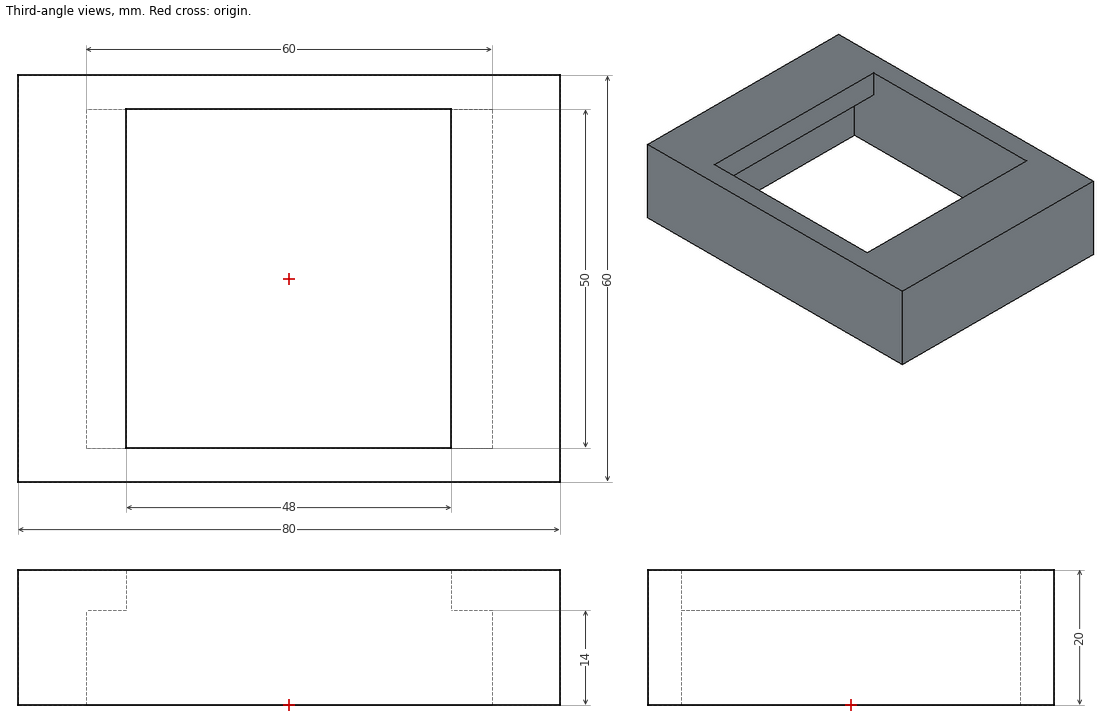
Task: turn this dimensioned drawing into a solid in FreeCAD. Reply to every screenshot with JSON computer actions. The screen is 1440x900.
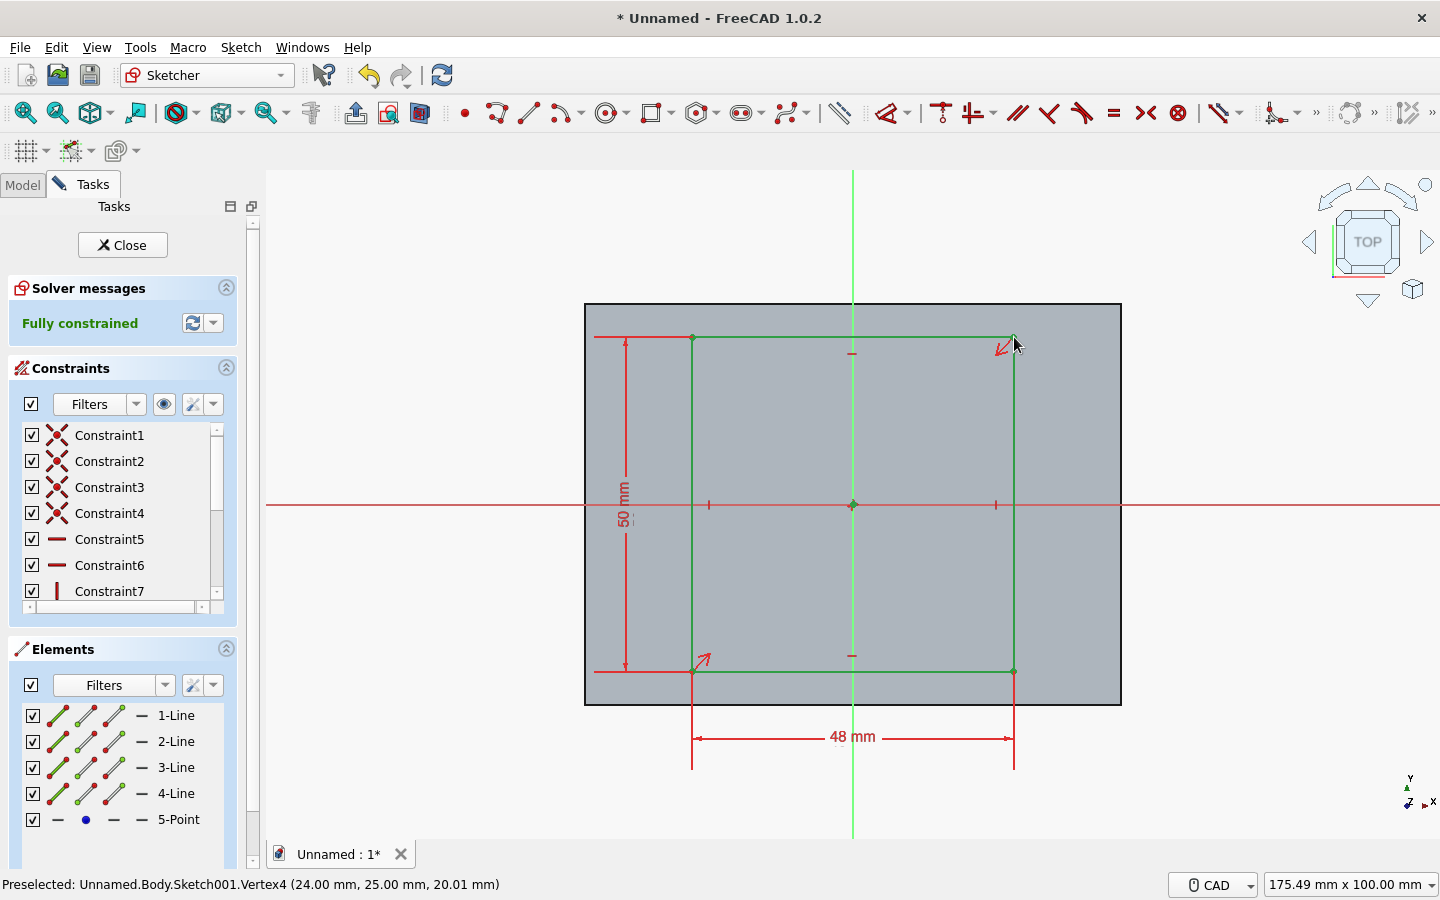
{"action": "left_click", "coordinate": [123, 245]}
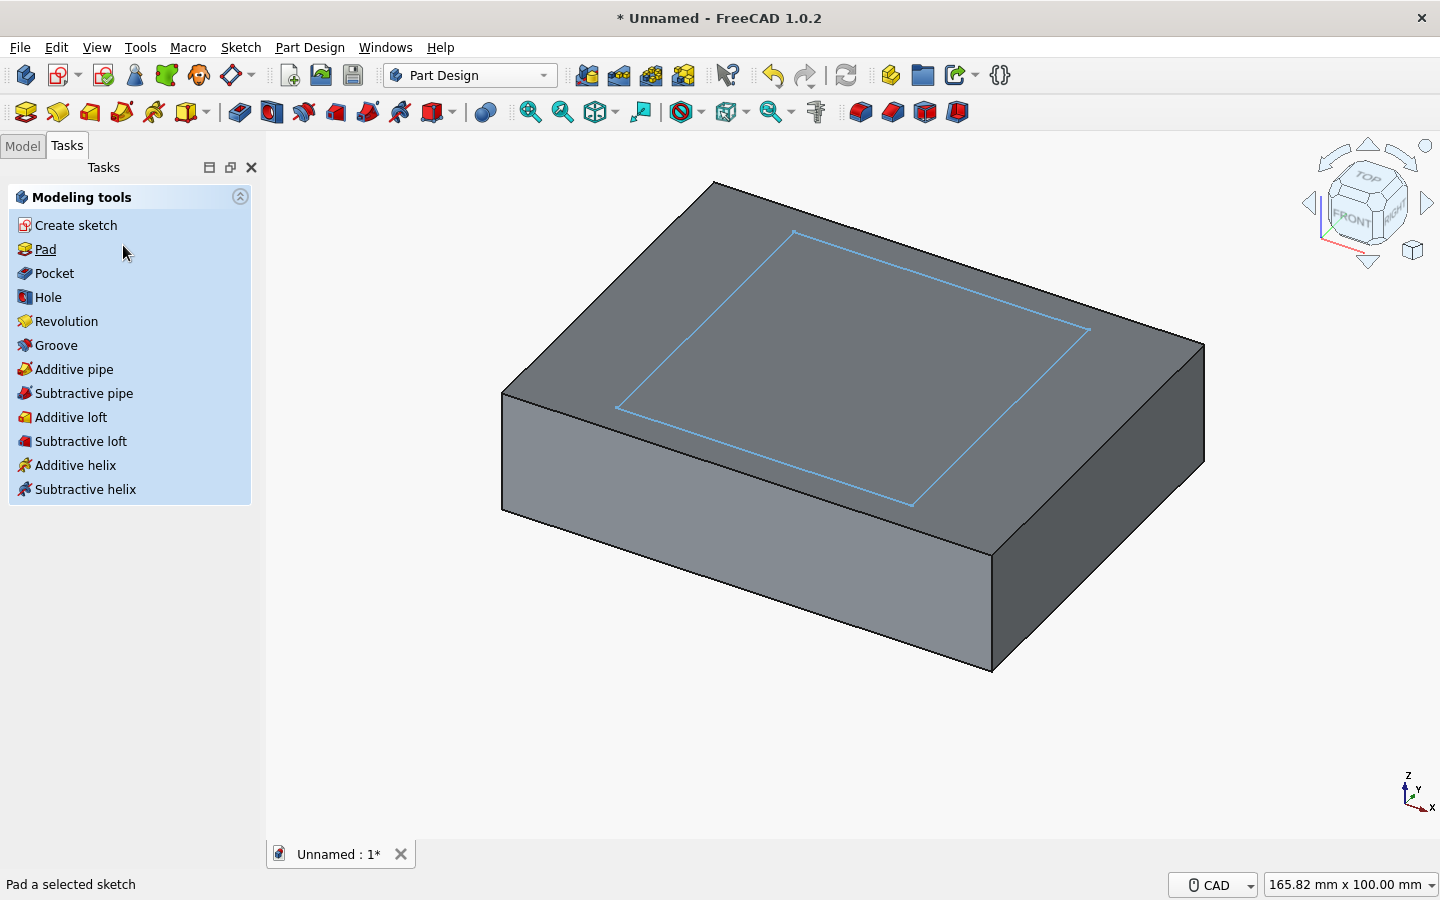
{"action": "left_click", "coordinate": [240, 112]}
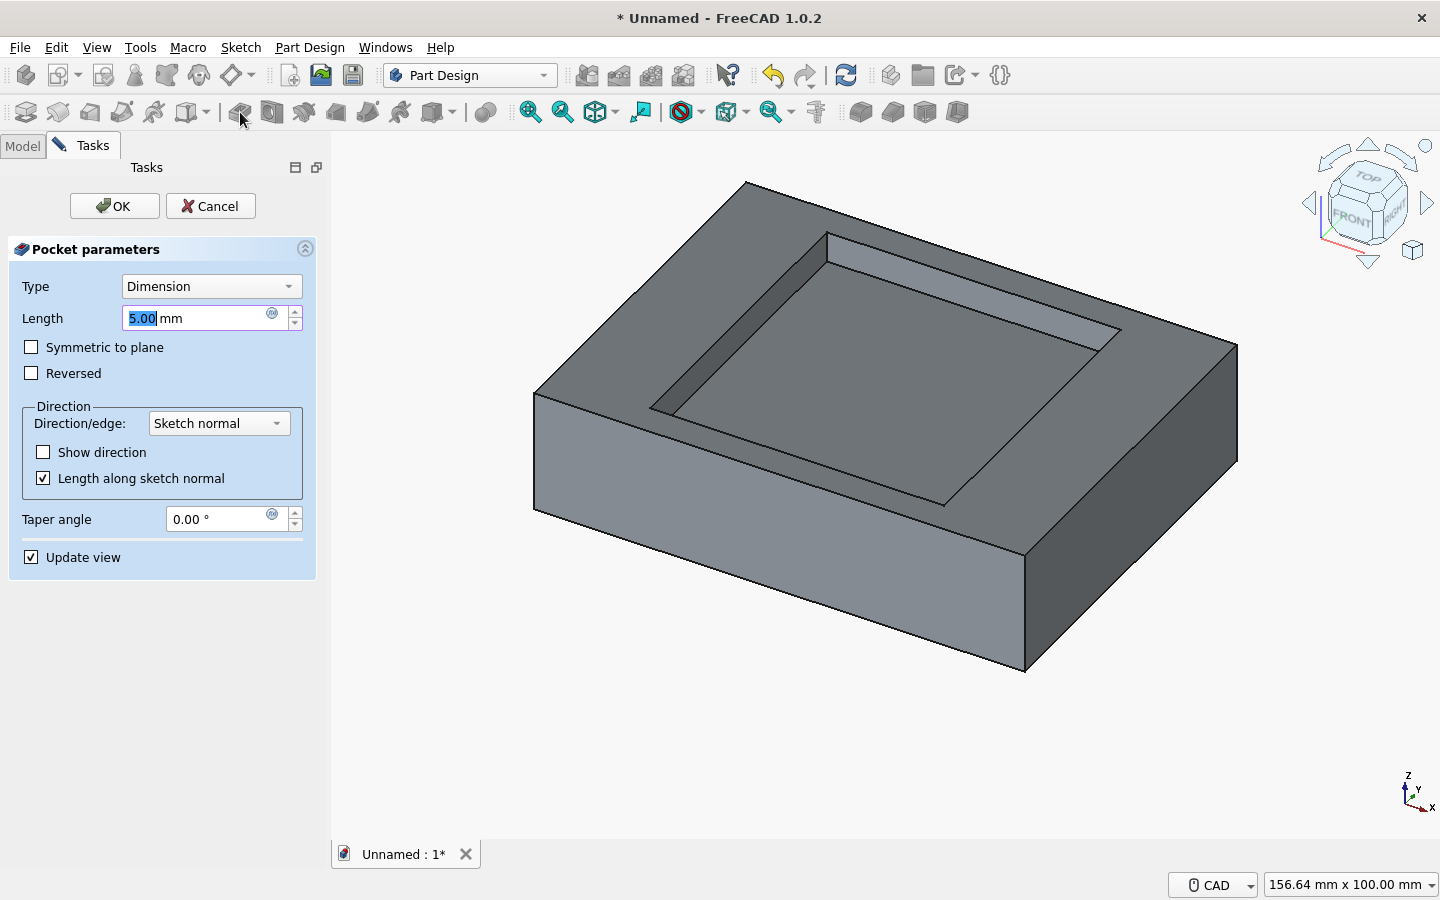
{"action": "left_click", "coordinate": [212, 286]}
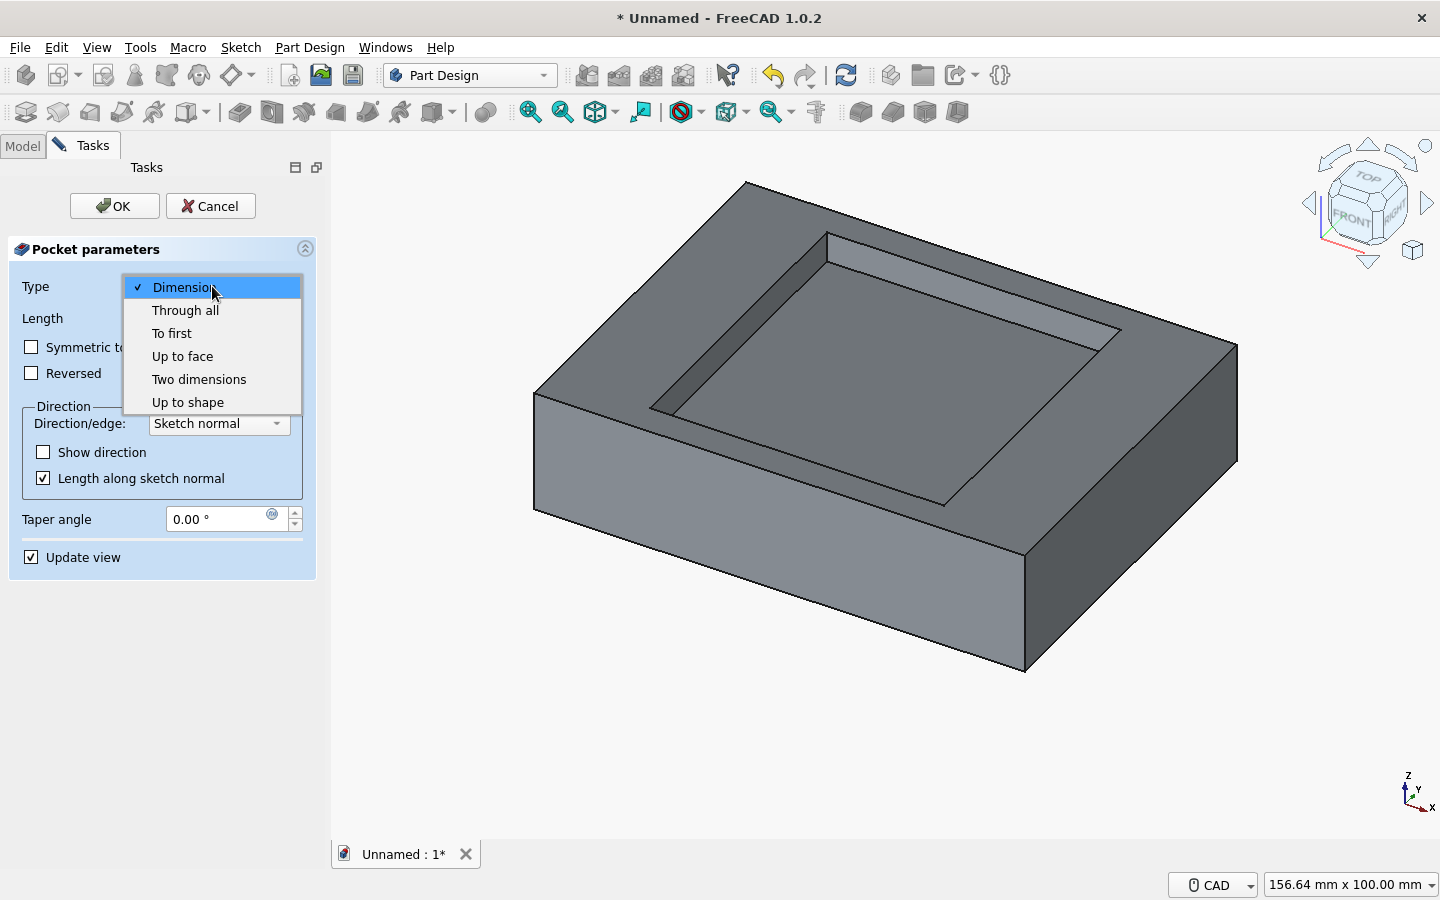
{"action": "left_click", "coordinate": [212, 334]}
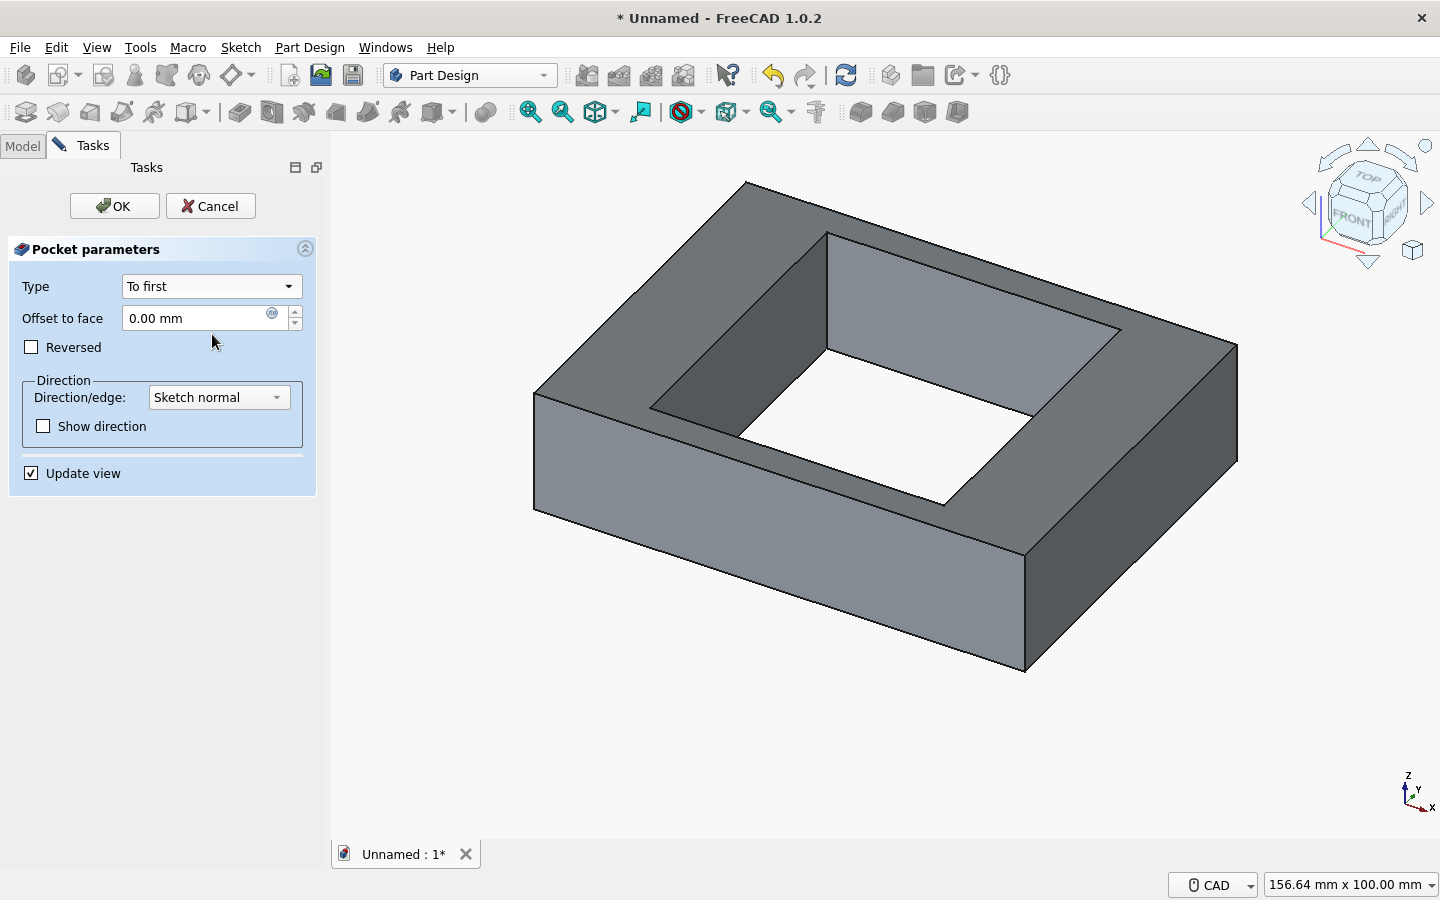
{"action": "left_click", "coordinate": [115, 206]}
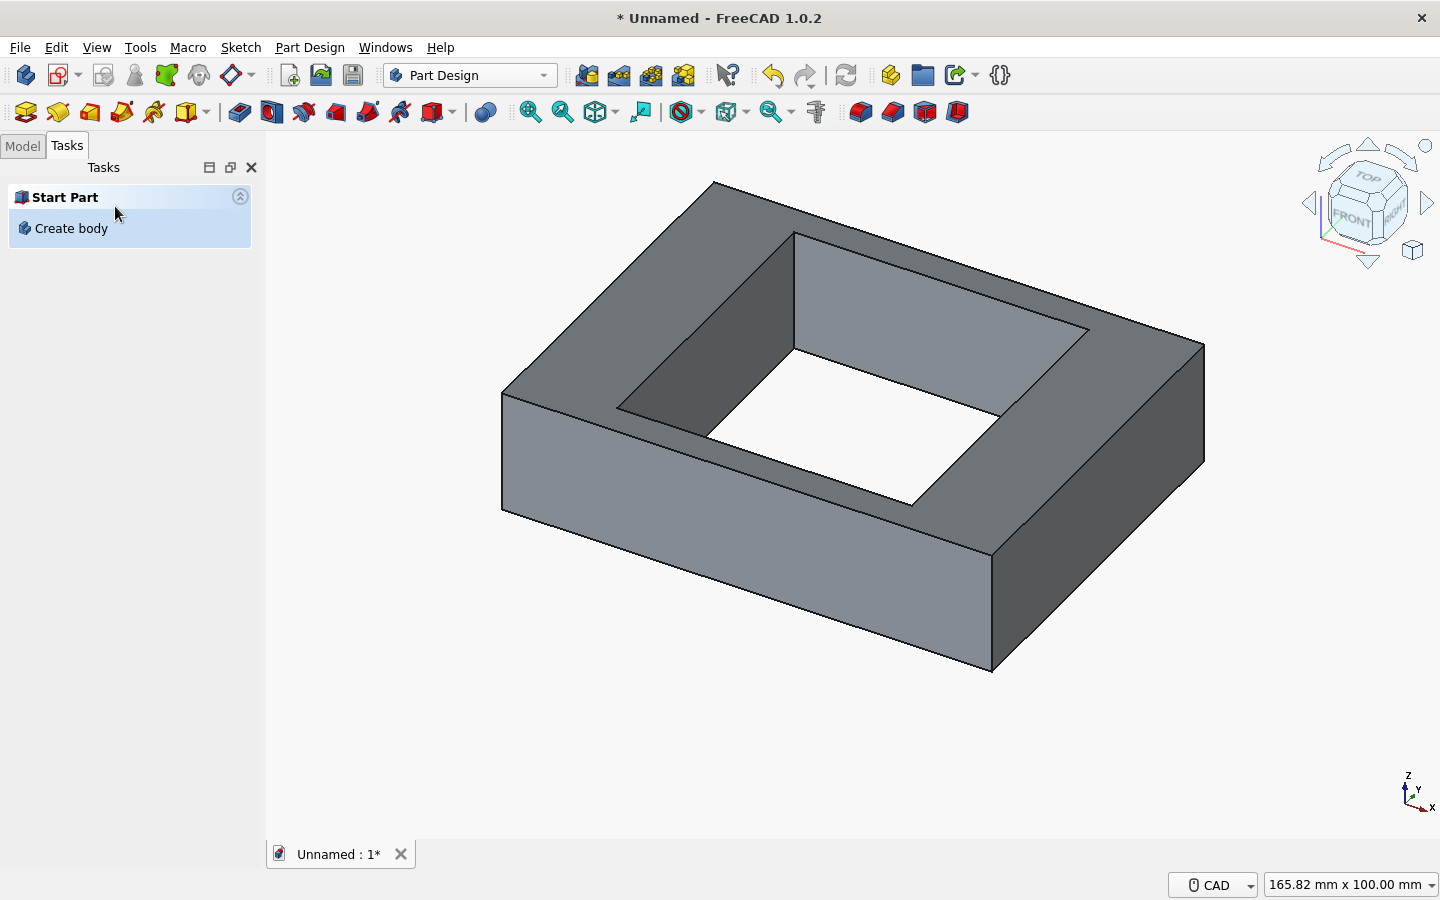
{"action": "key", "text": "5"}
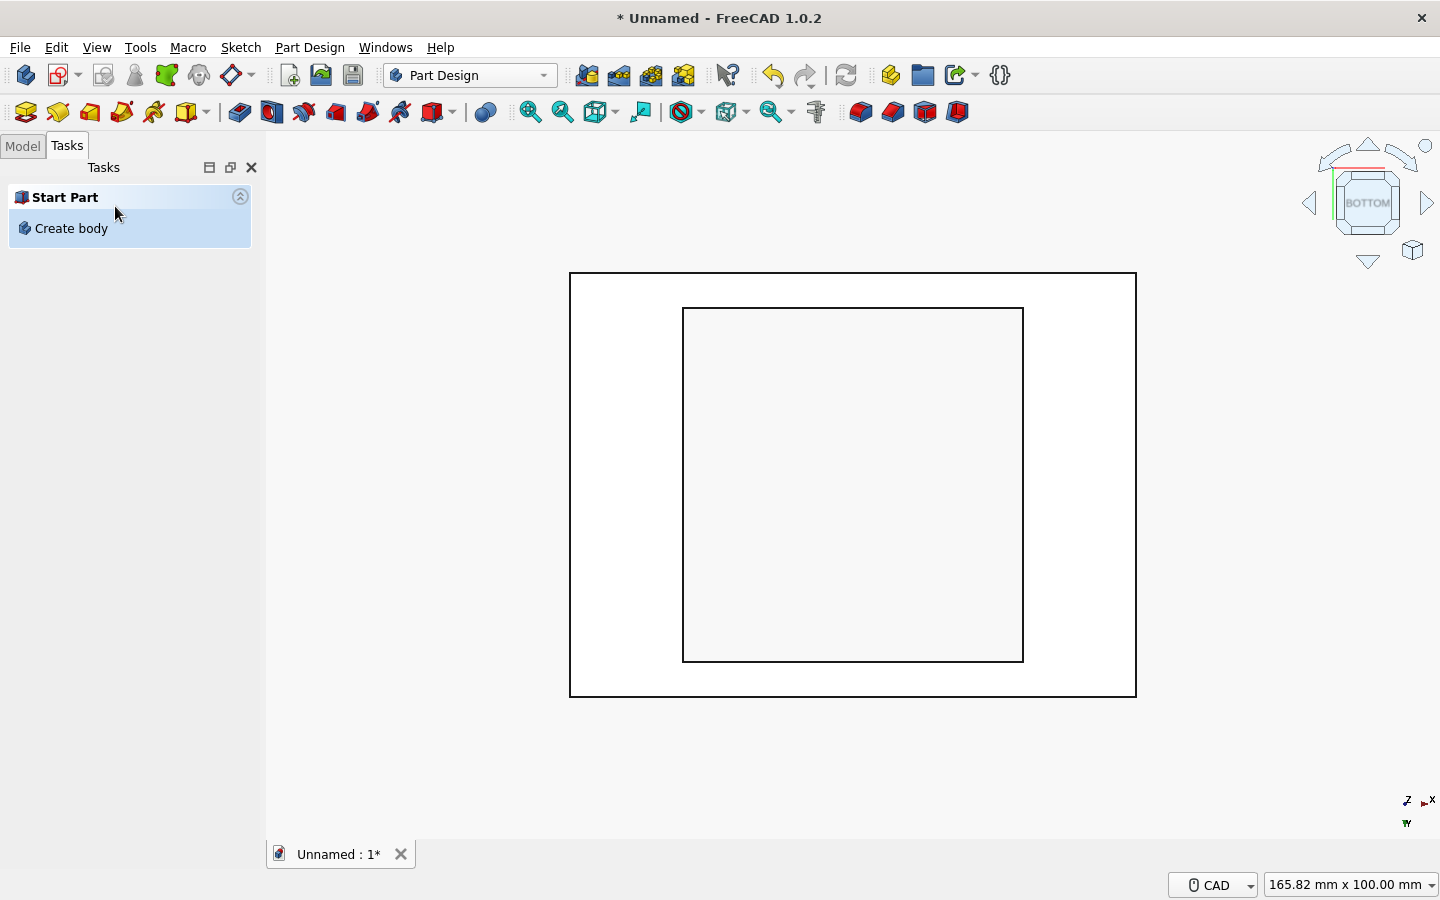
{"action": "left_click", "coordinate": [610, 605]}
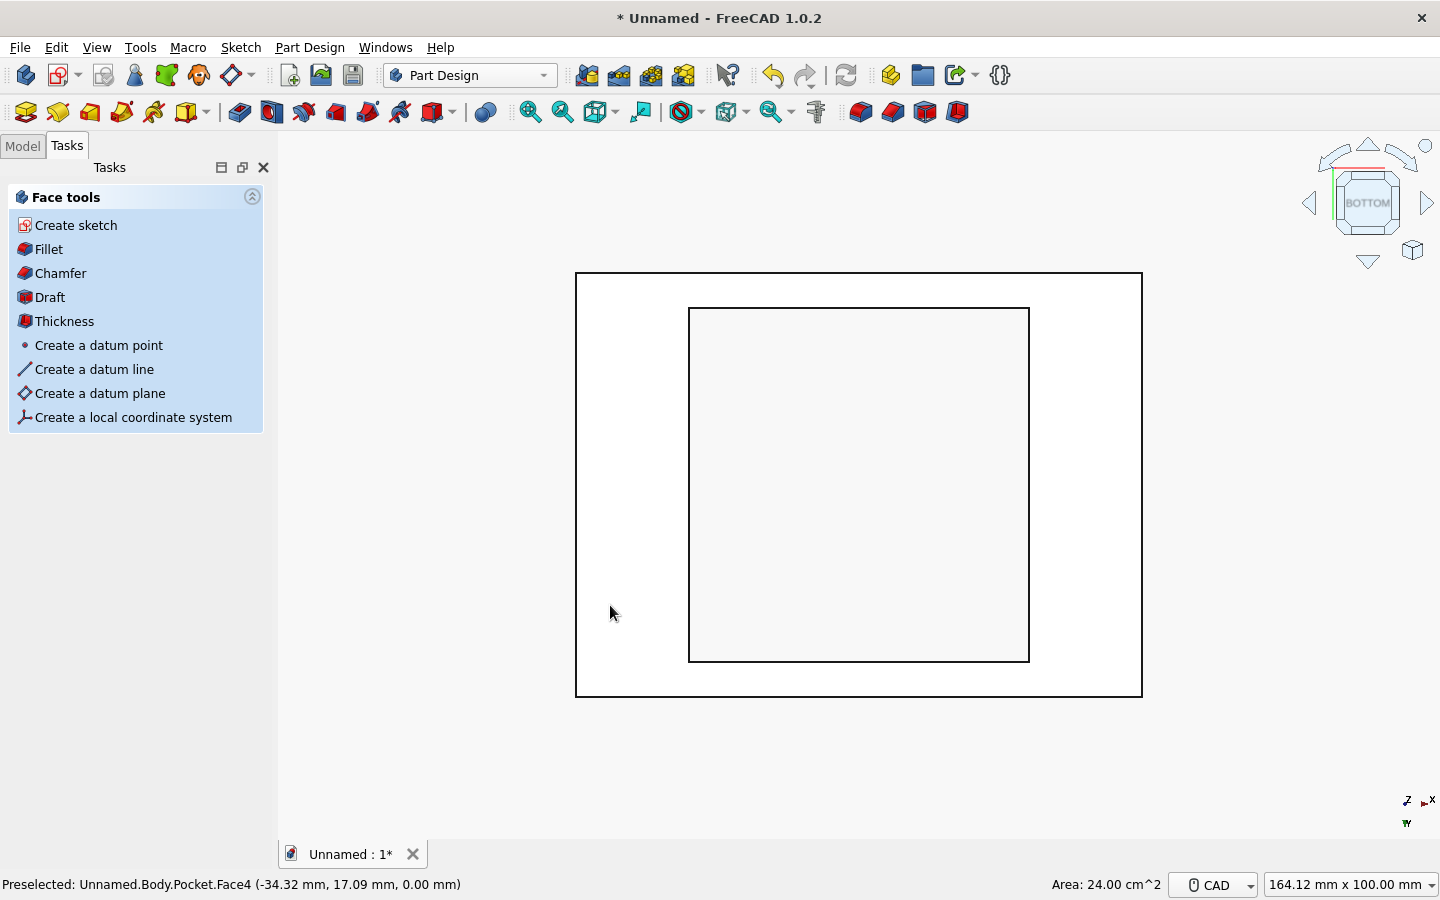
{"action": "left_click", "coordinate": [58, 76]}